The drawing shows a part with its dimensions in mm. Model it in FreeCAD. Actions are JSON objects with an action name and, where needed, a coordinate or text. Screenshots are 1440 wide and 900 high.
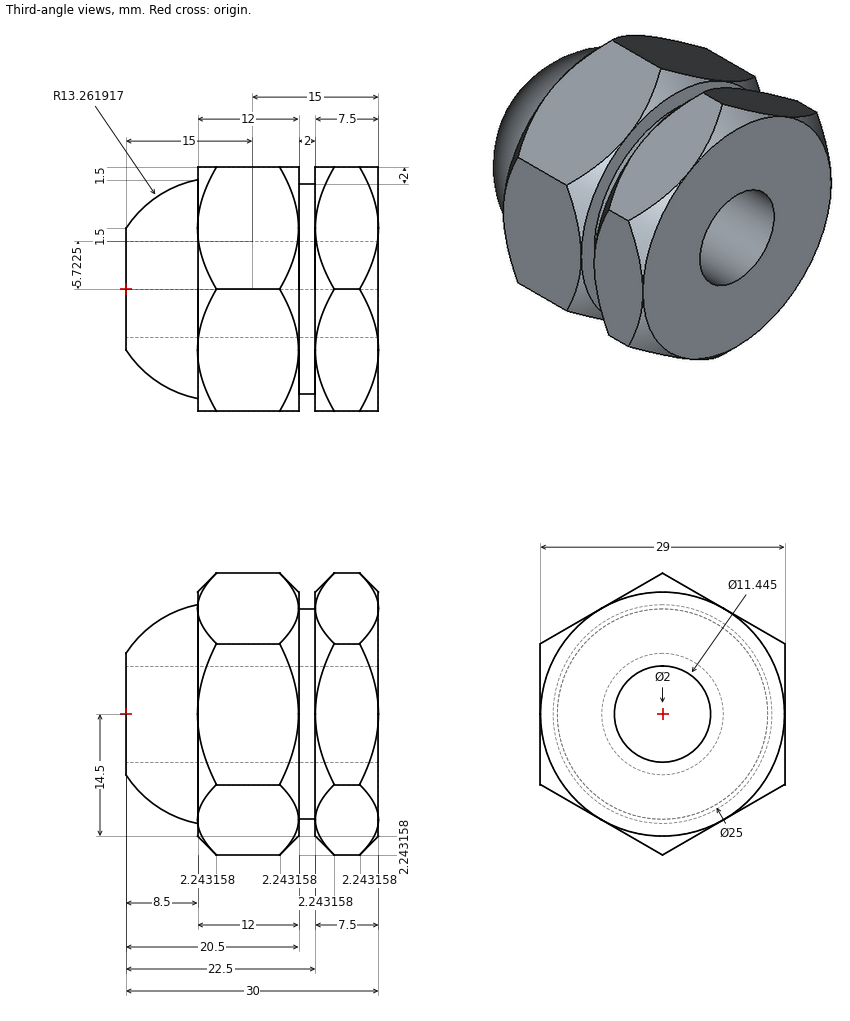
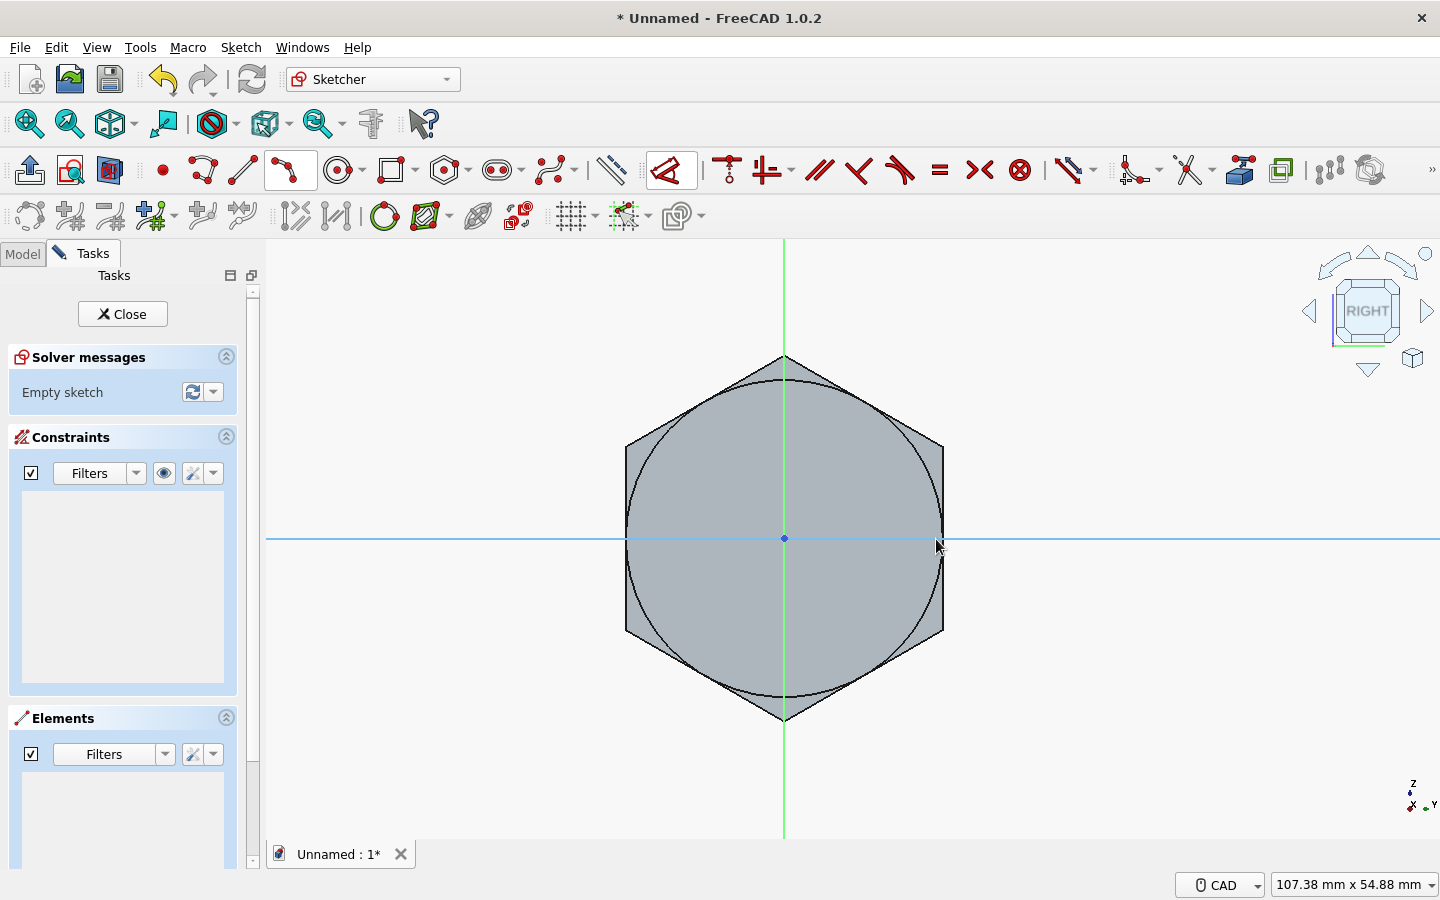
{"action": "key", "text": "g p 6"}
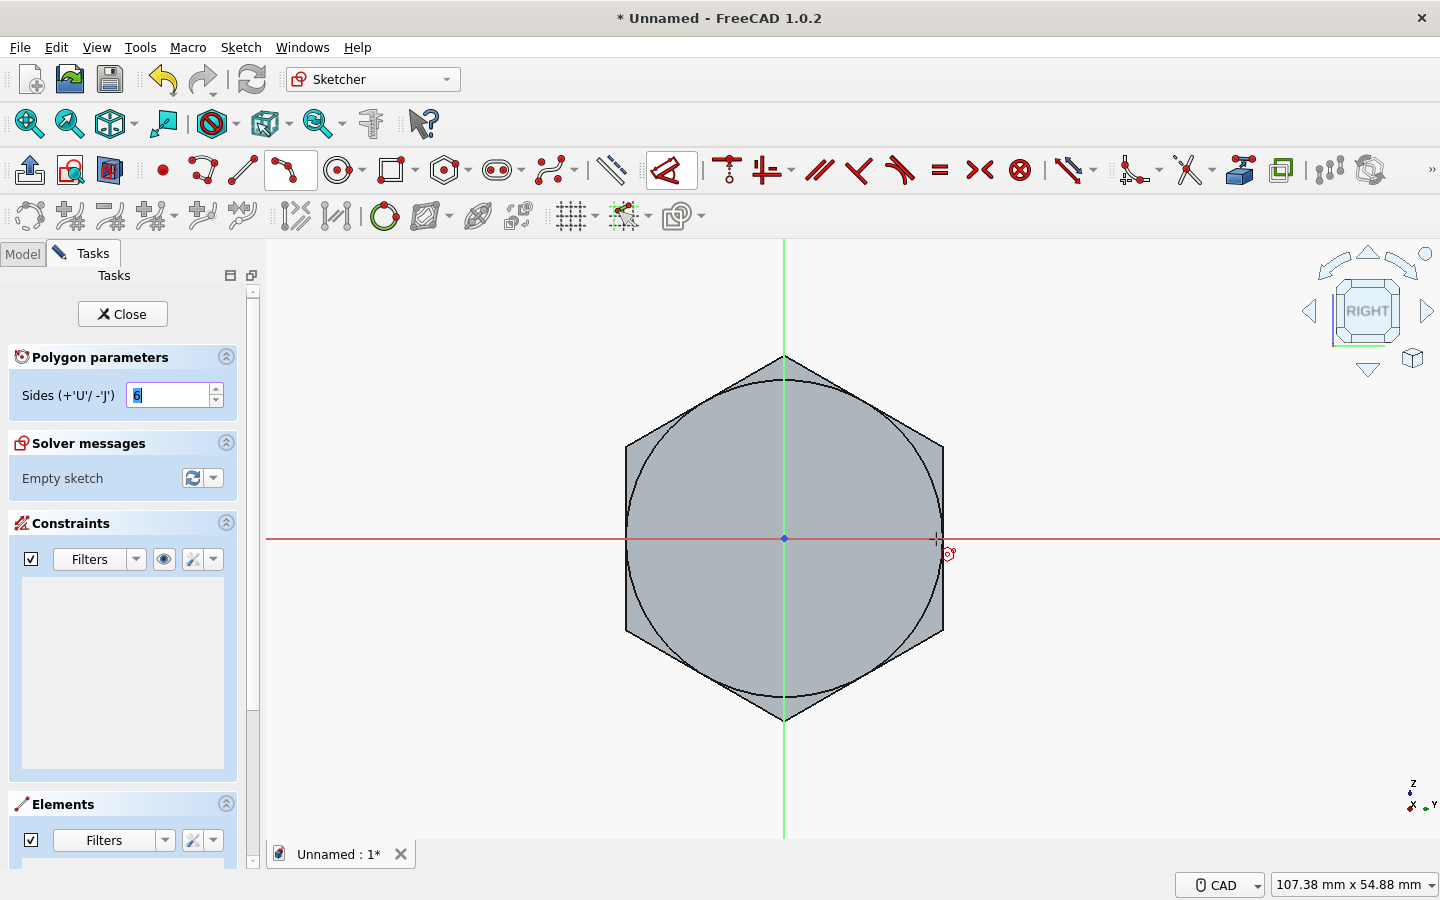
{"action": "left_click", "coordinate": [784, 539]}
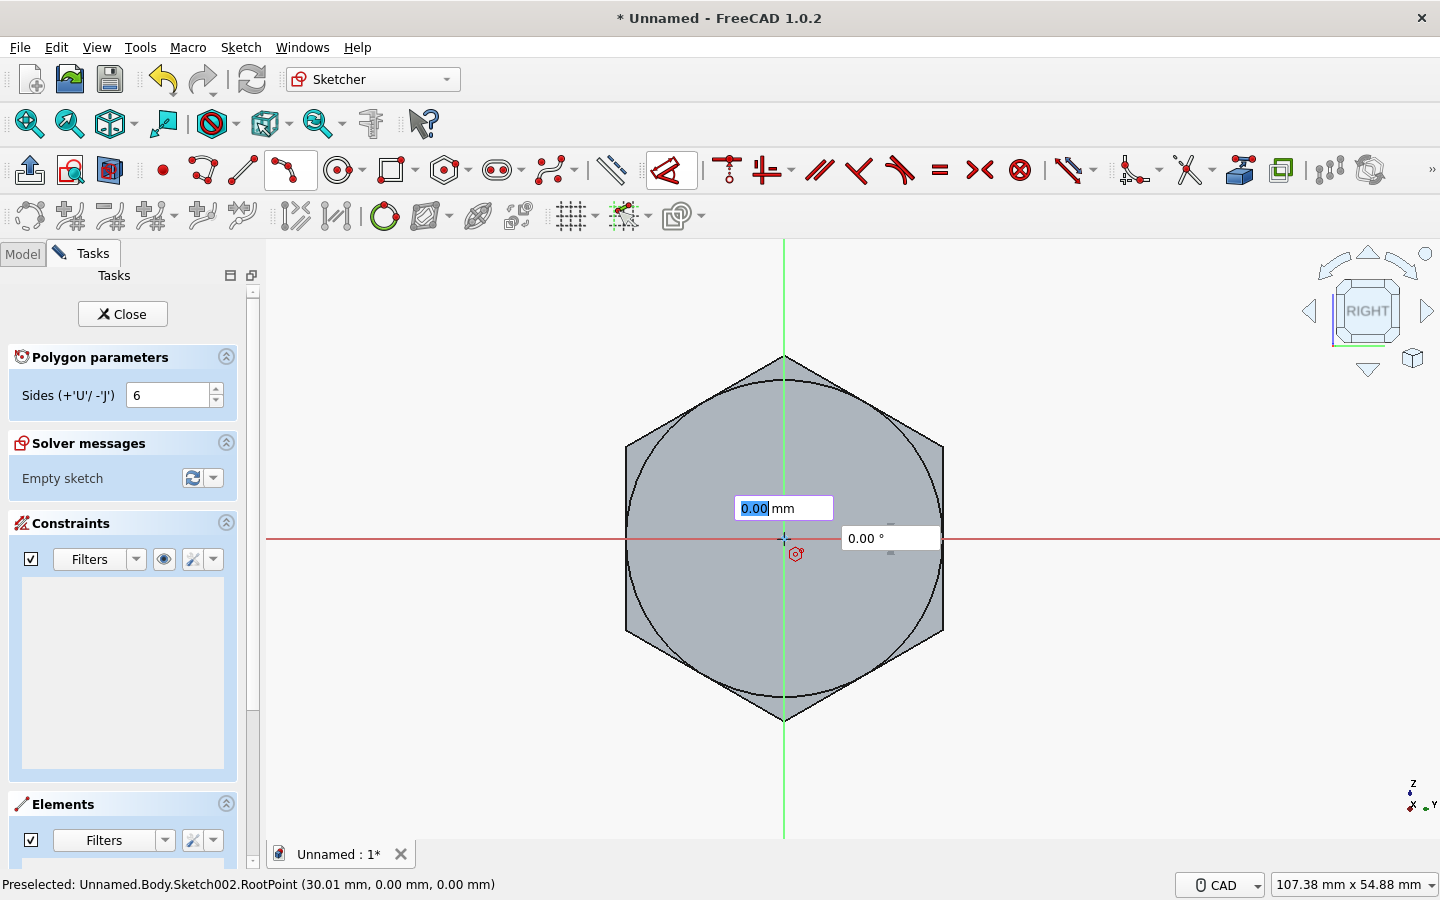
{"action": "left_click", "coordinate": [784, 722]}
{"action": "key", "text": "Escape"}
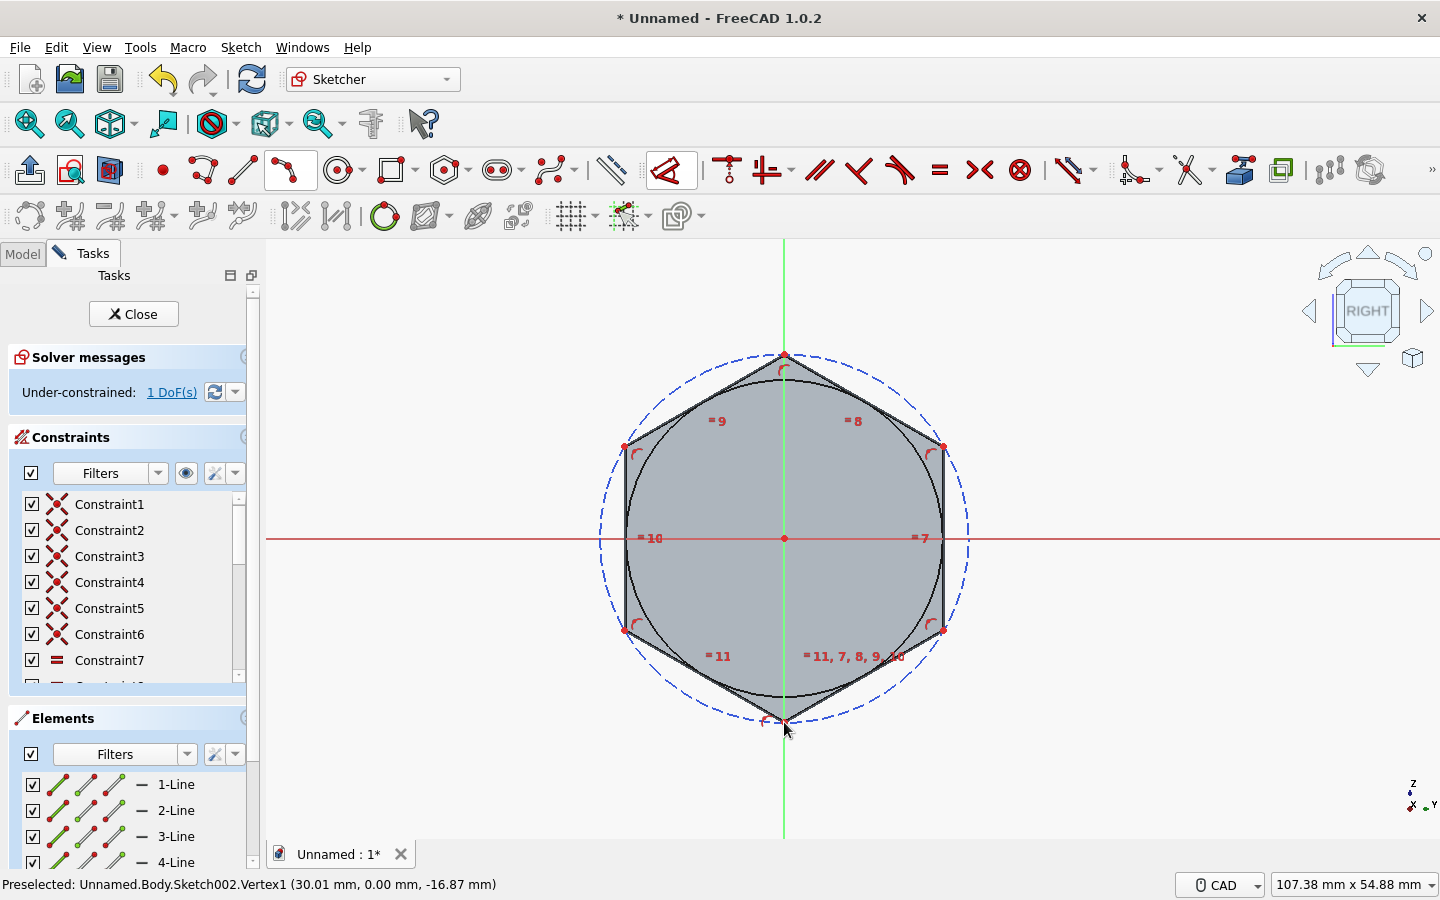
{"action": "left_click", "coordinate": [338, 170]}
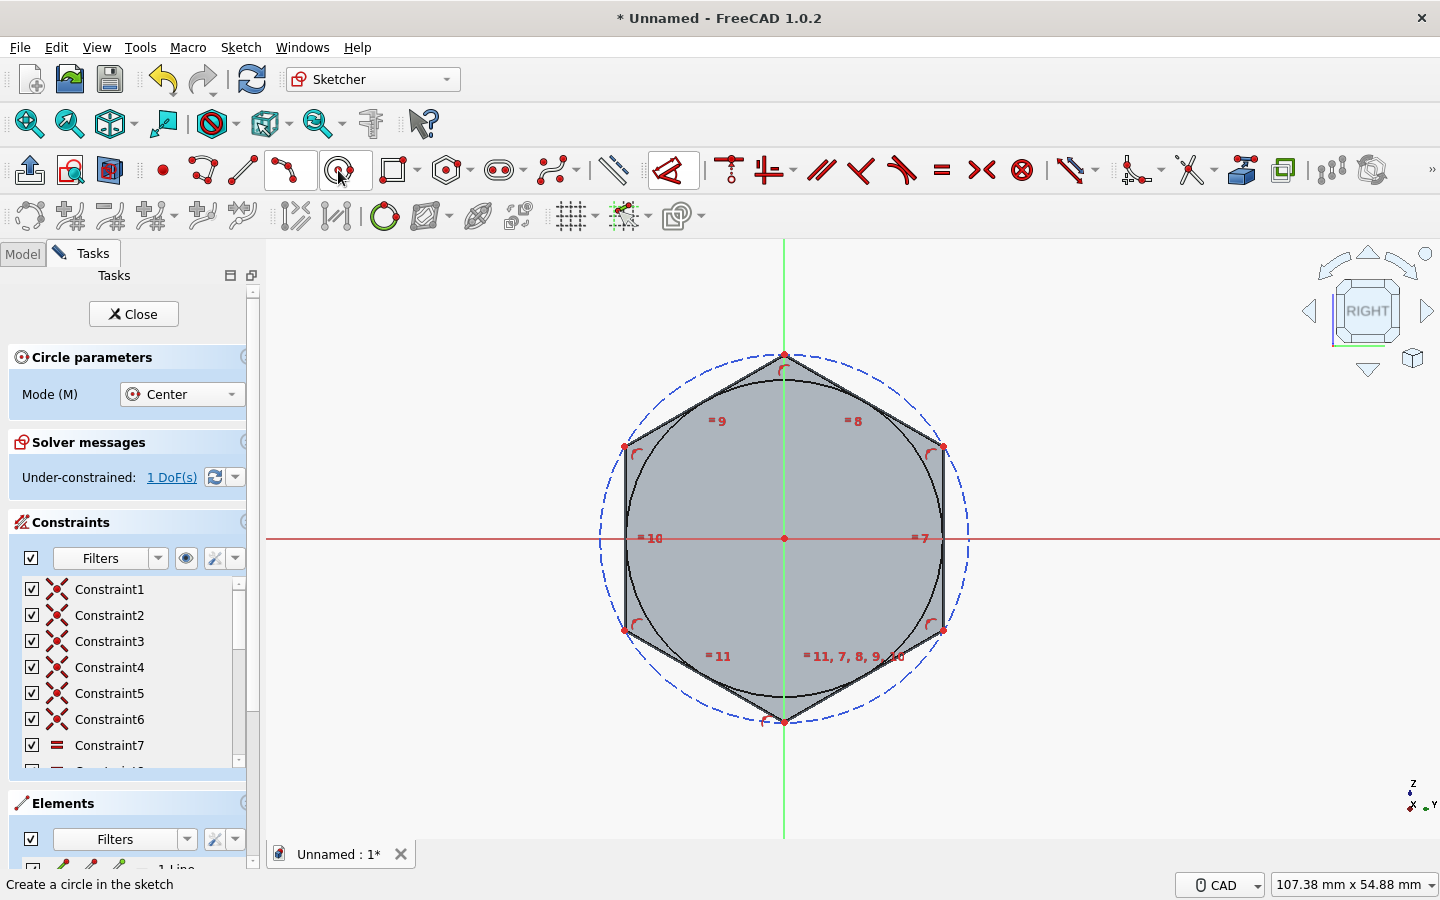
{"action": "left_click", "coordinate": [784, 539]}
{"action": "left_click", "coordinate": [881, 442]}
{"action": "key", "text": "Escape"}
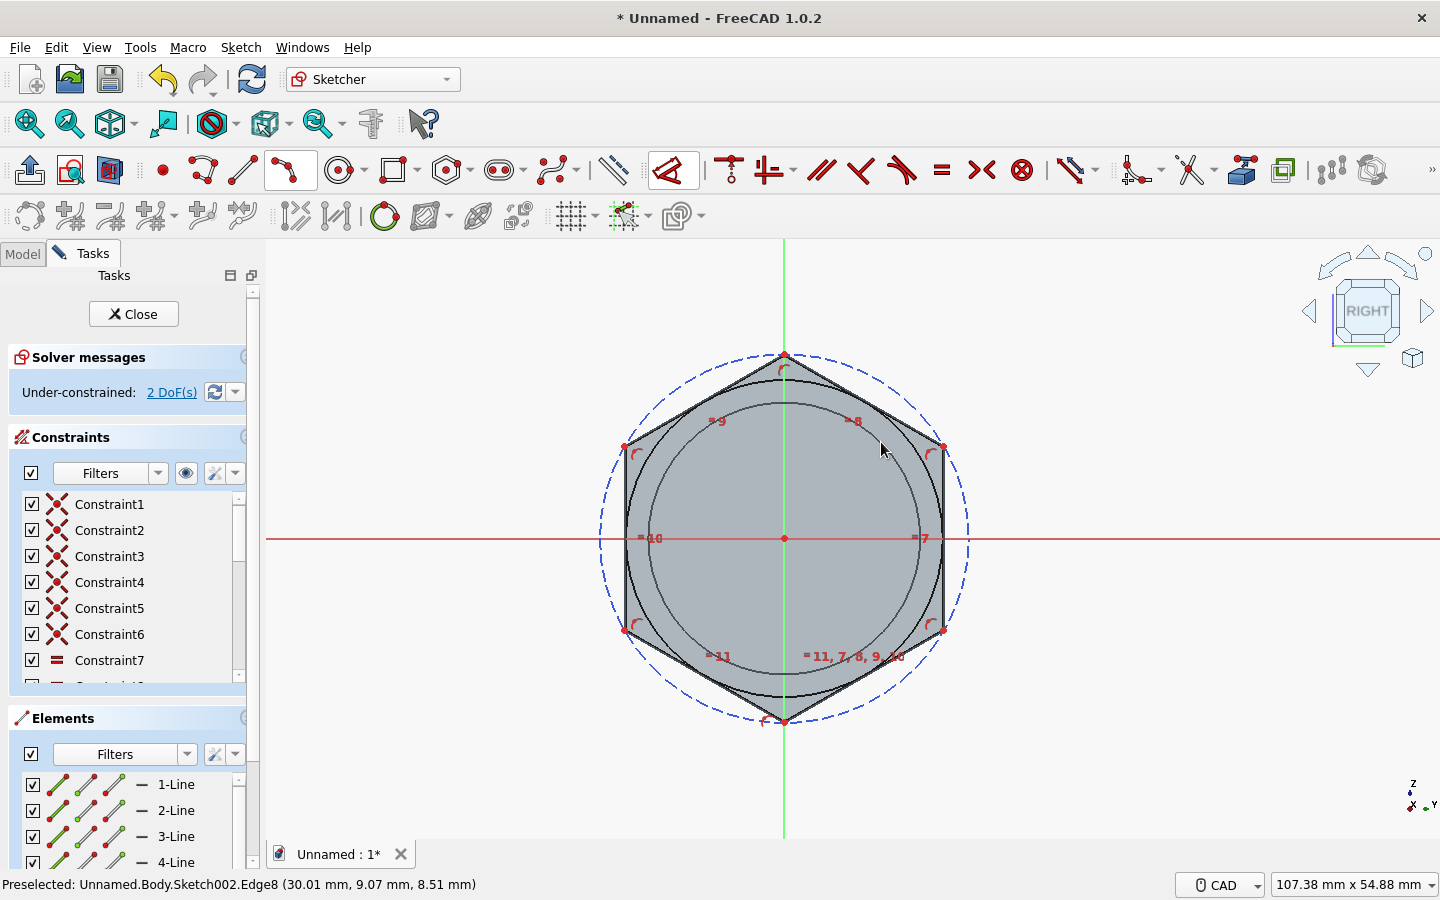
{"action": "left_click", "coordinate": [880, 442]}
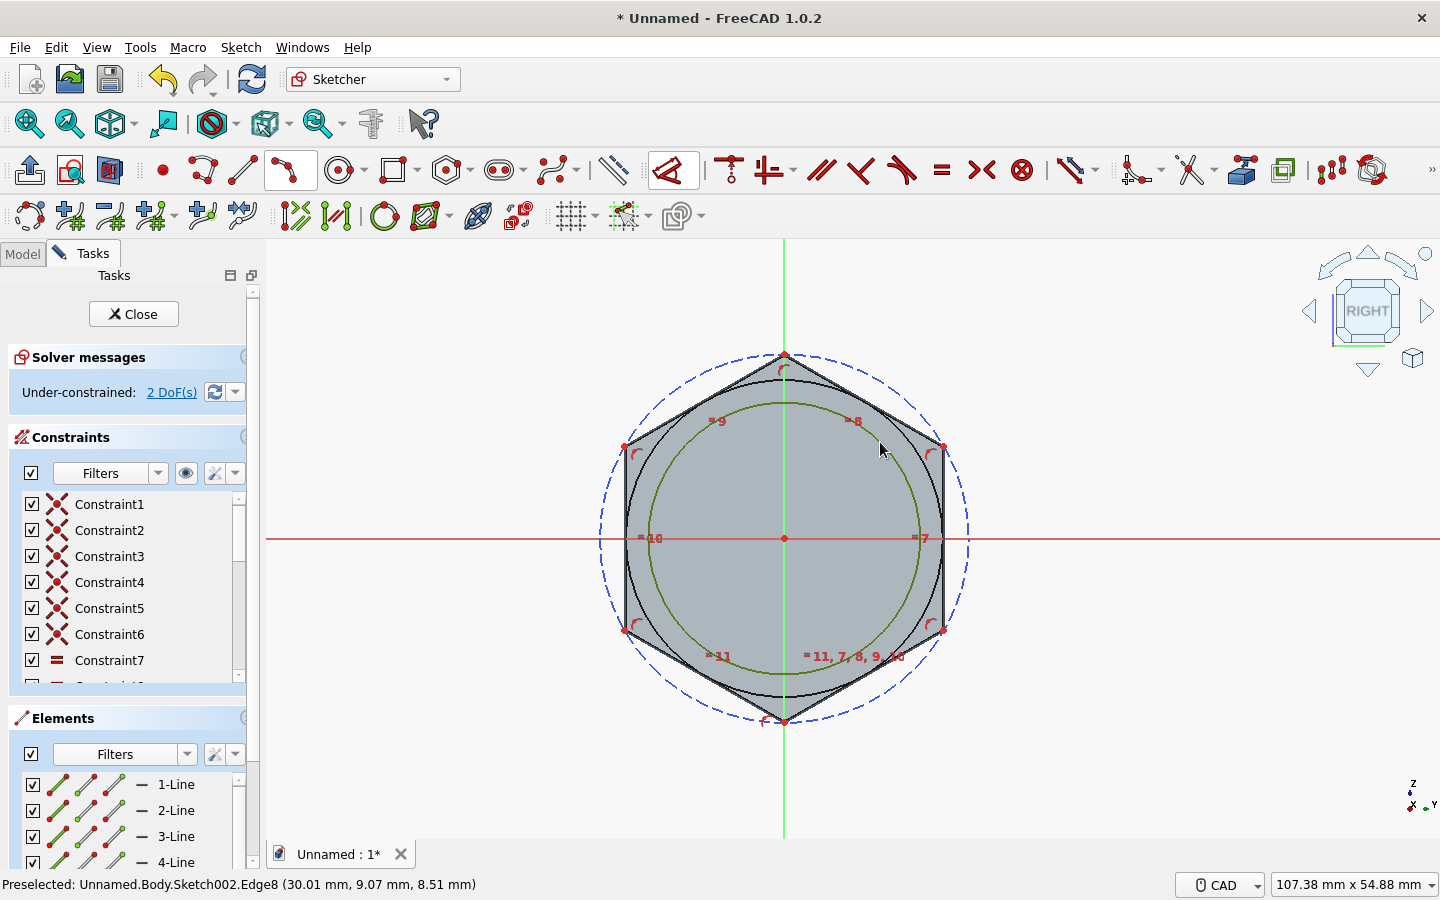
{"action": "key", "text": "k o"}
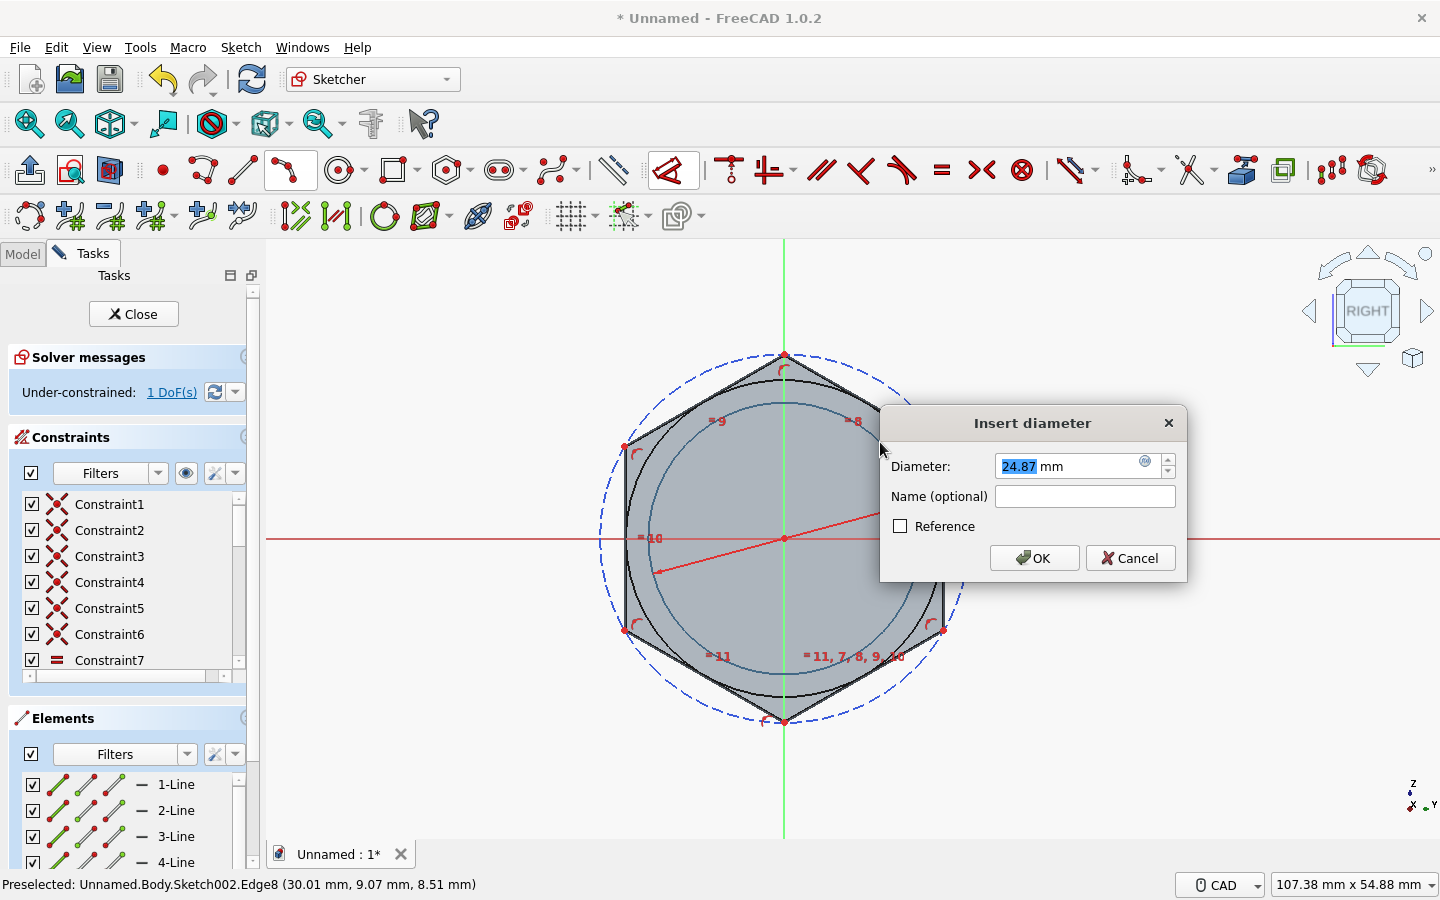
{"action": "type", "text": "25"}
{"action": "key", "text": "Return"}